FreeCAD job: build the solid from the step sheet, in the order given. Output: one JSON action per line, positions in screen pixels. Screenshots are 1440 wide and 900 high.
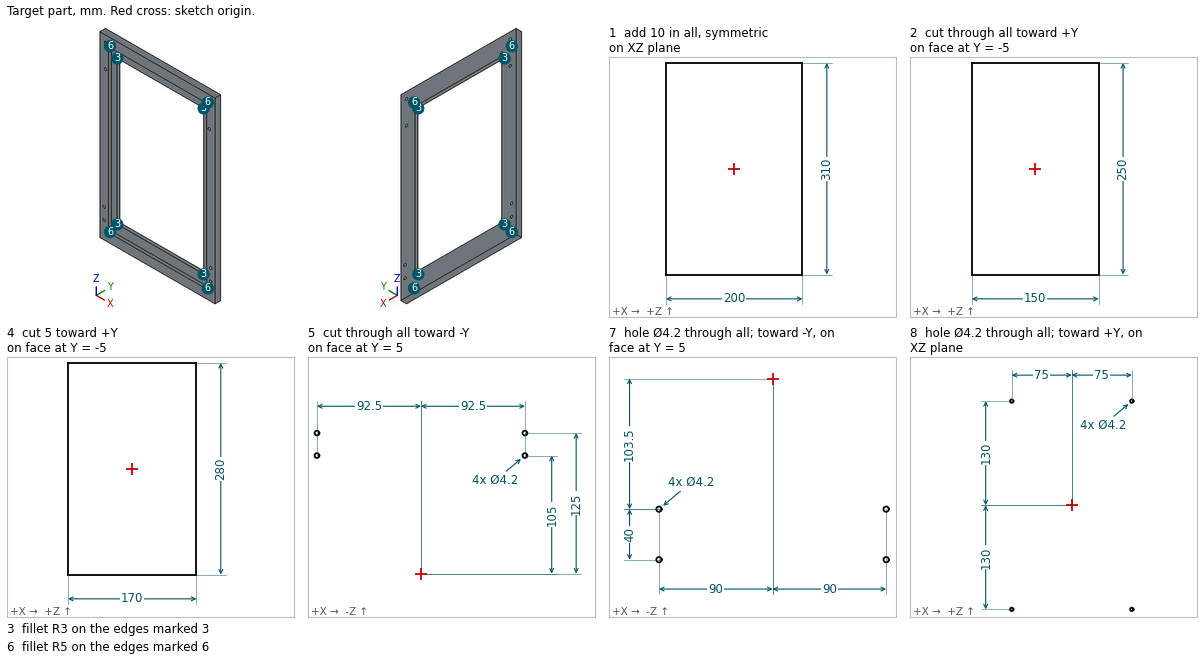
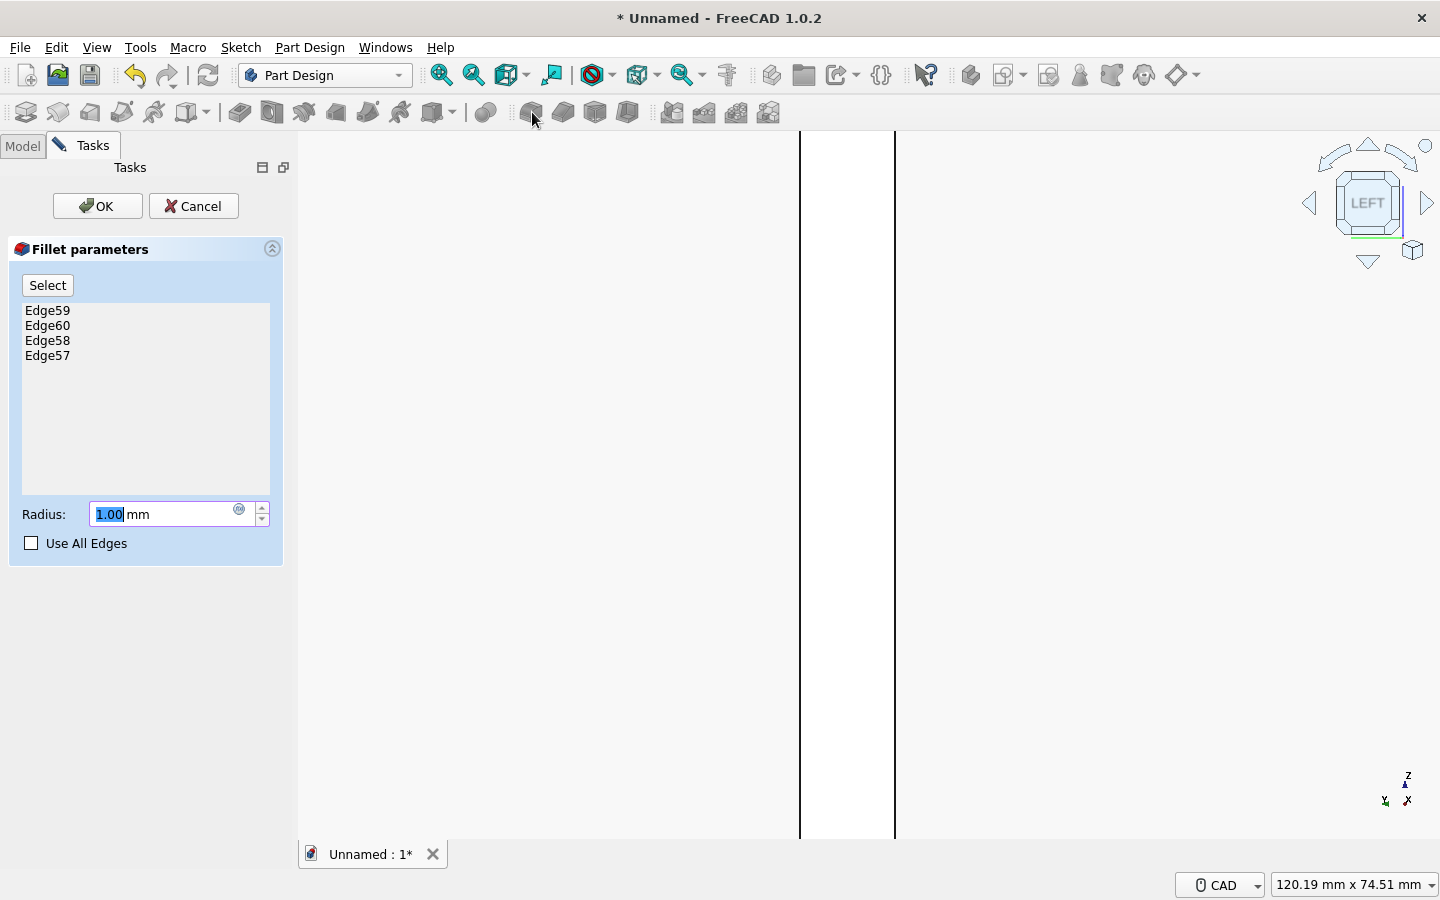
{"action": "type", "text": "5"}
{"action": "key", "text": "Tab"}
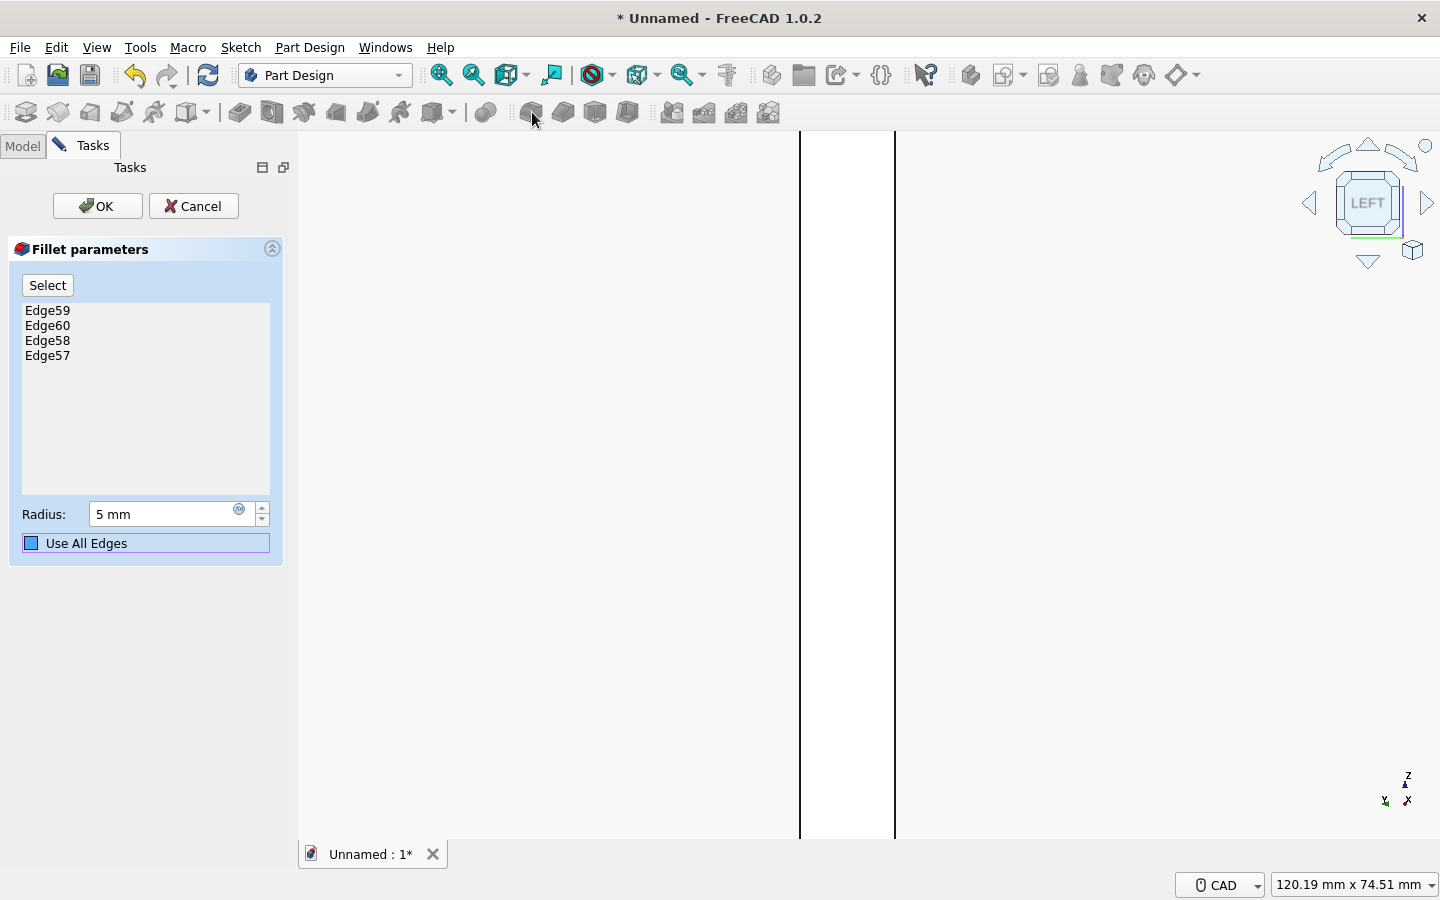
{"action": "left_click", "coordinate": [98, 206]}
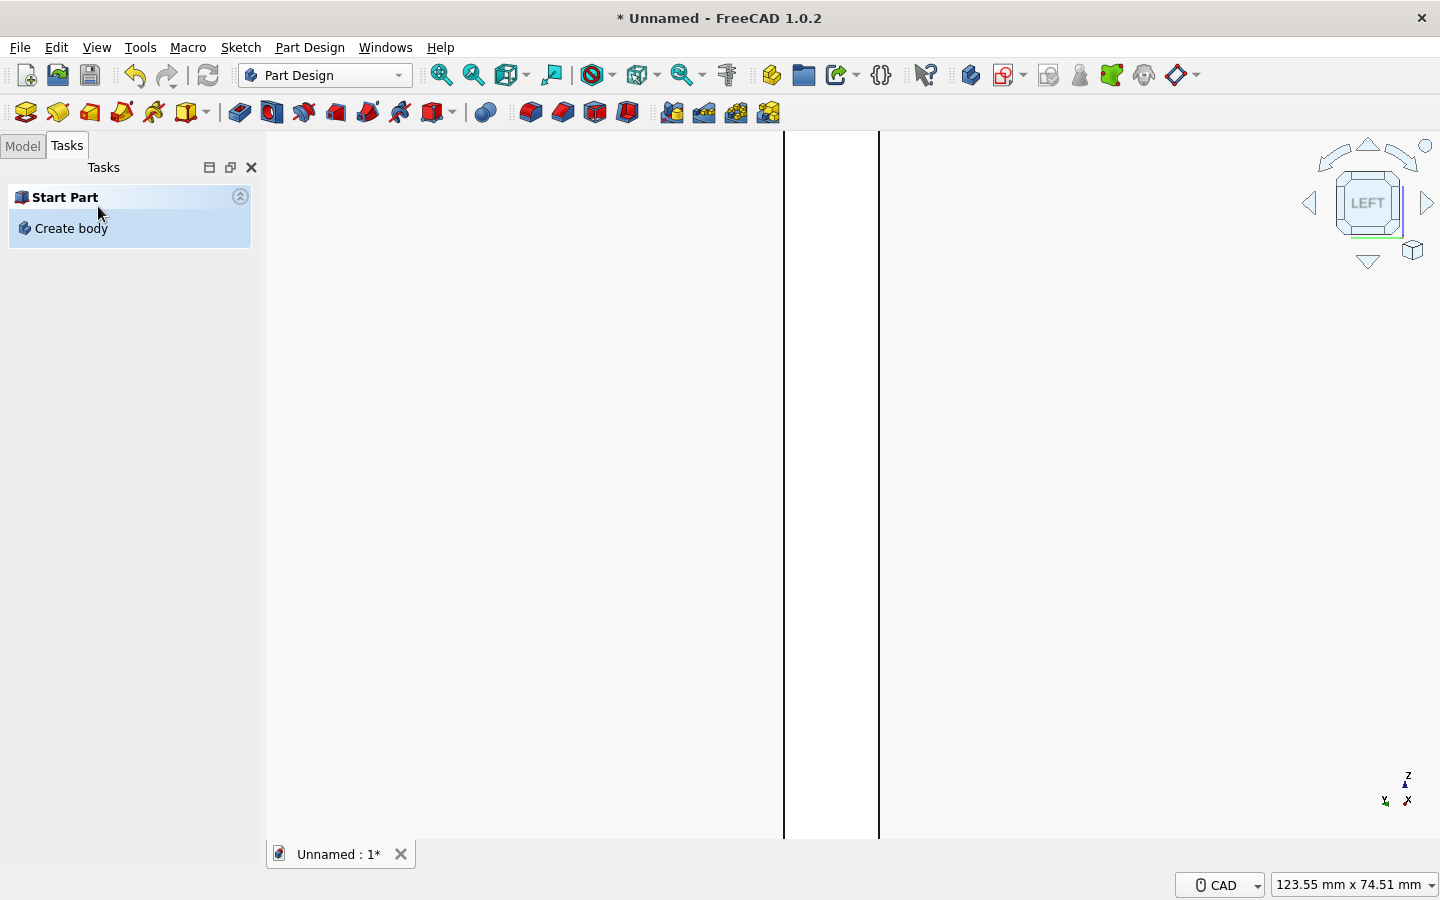
{"action": "key", "text": "v f"}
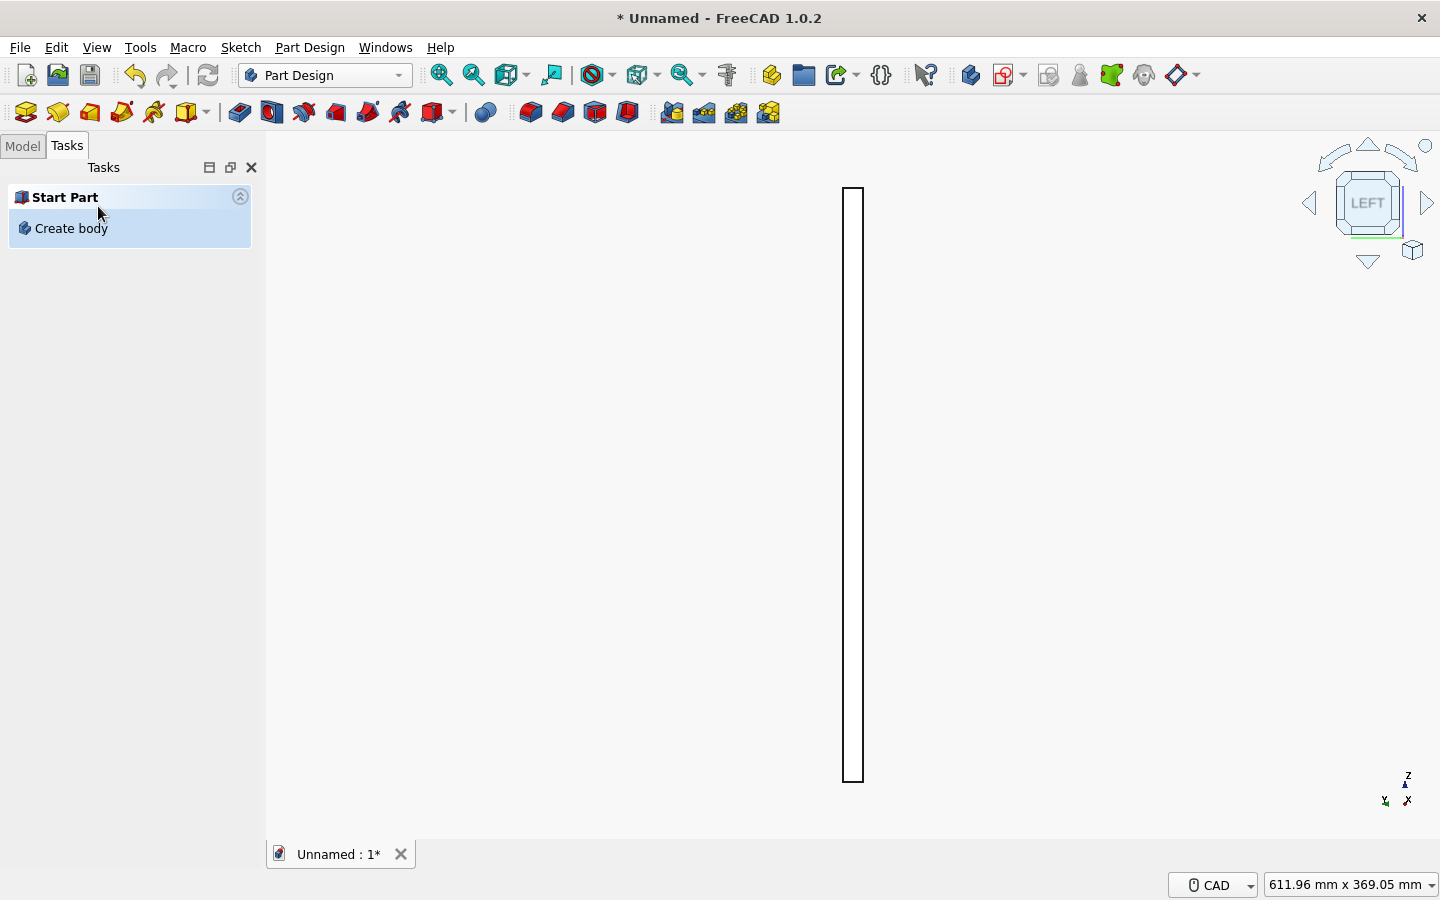
{"action": "key", "text": "4"}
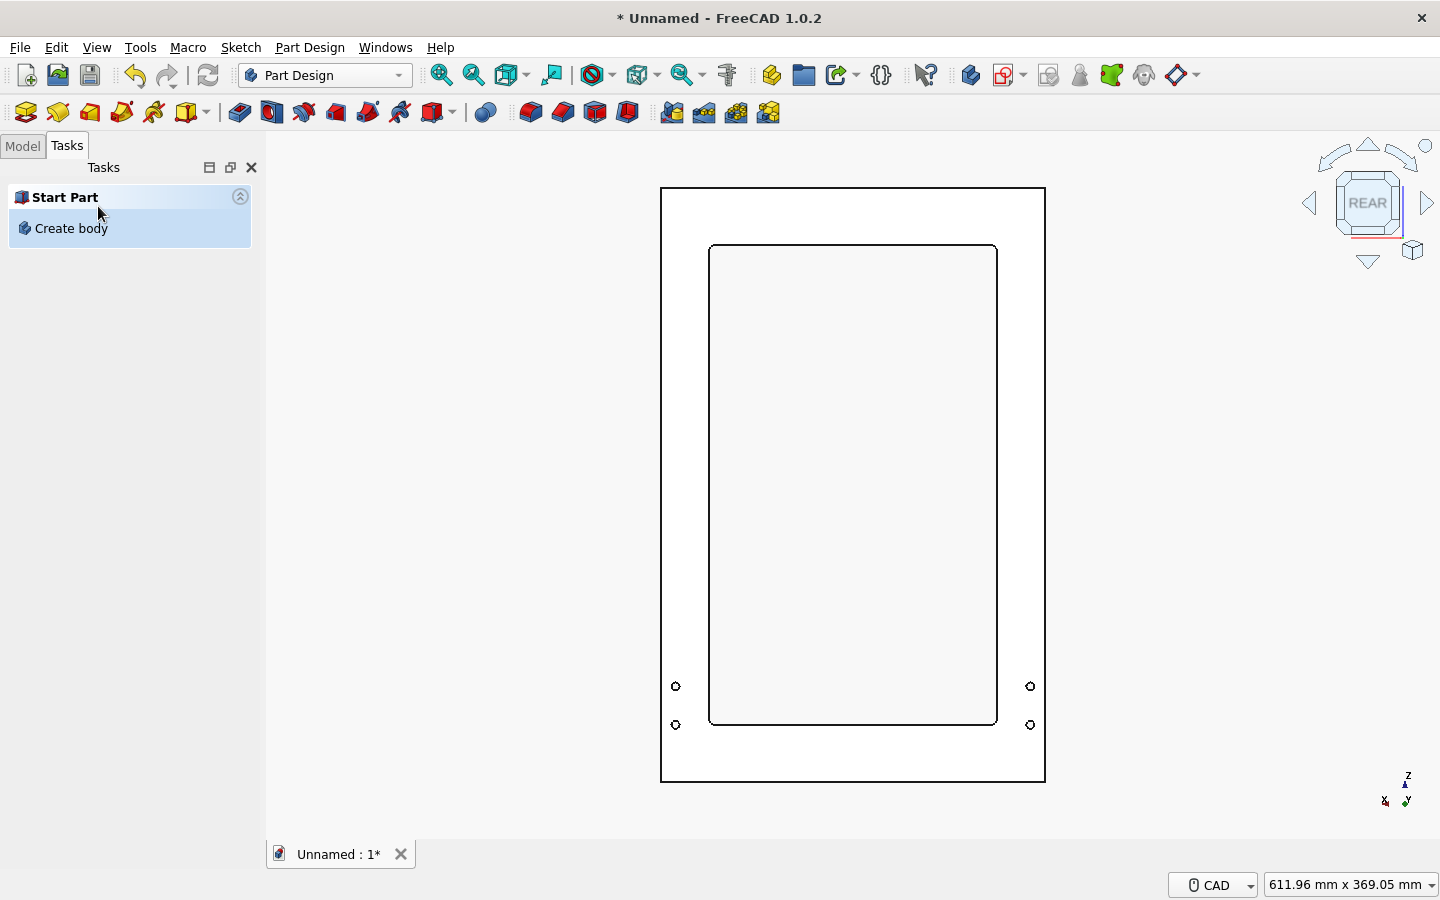
{"action": "left_click", "coordinate": [1017, 229]}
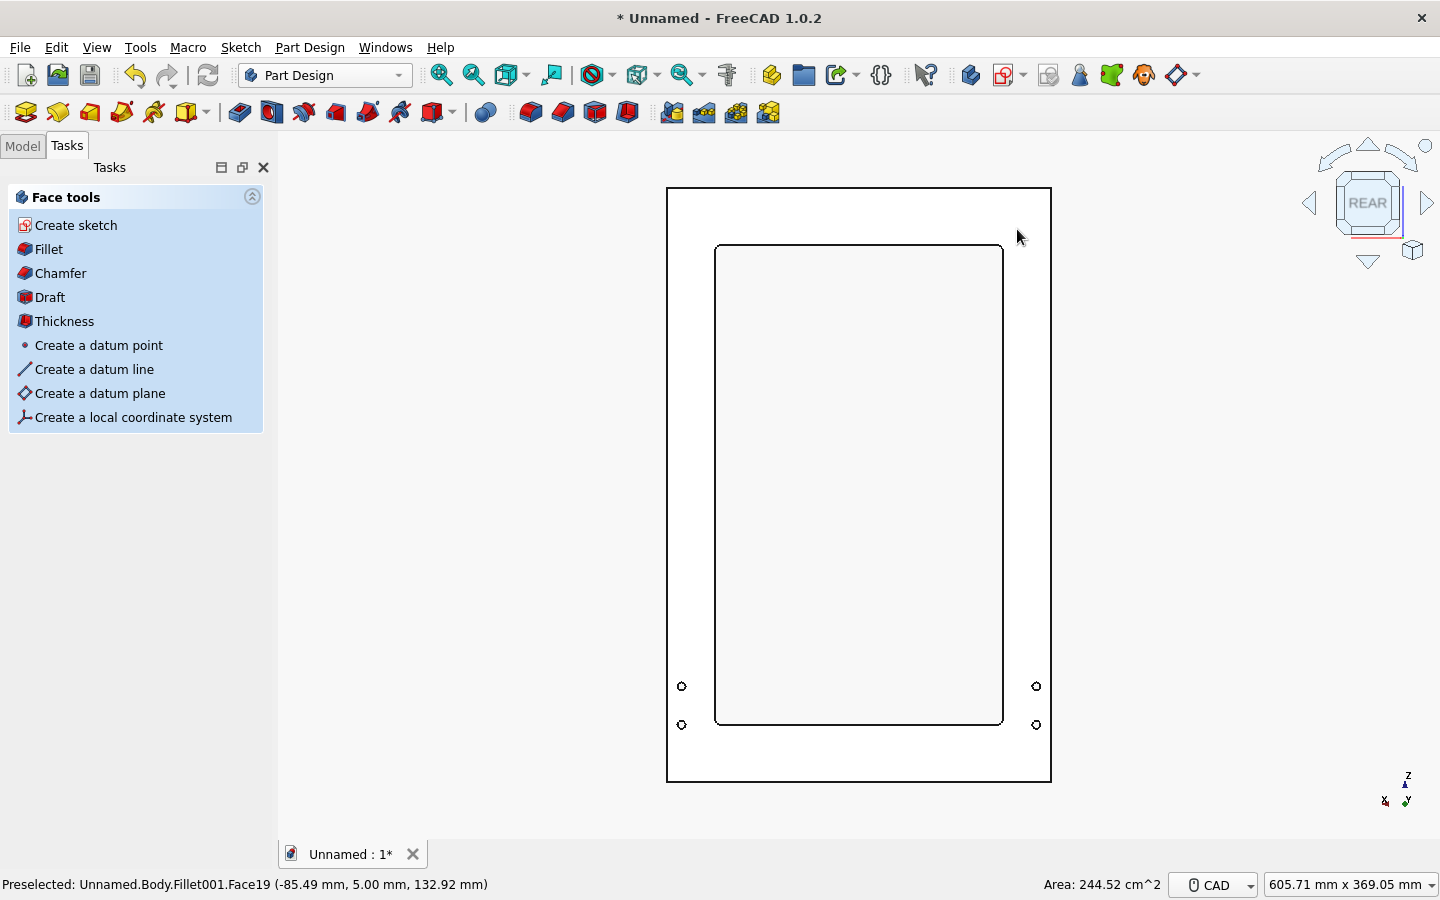
{"action": "left_click", "coordinate": [1004, 76]}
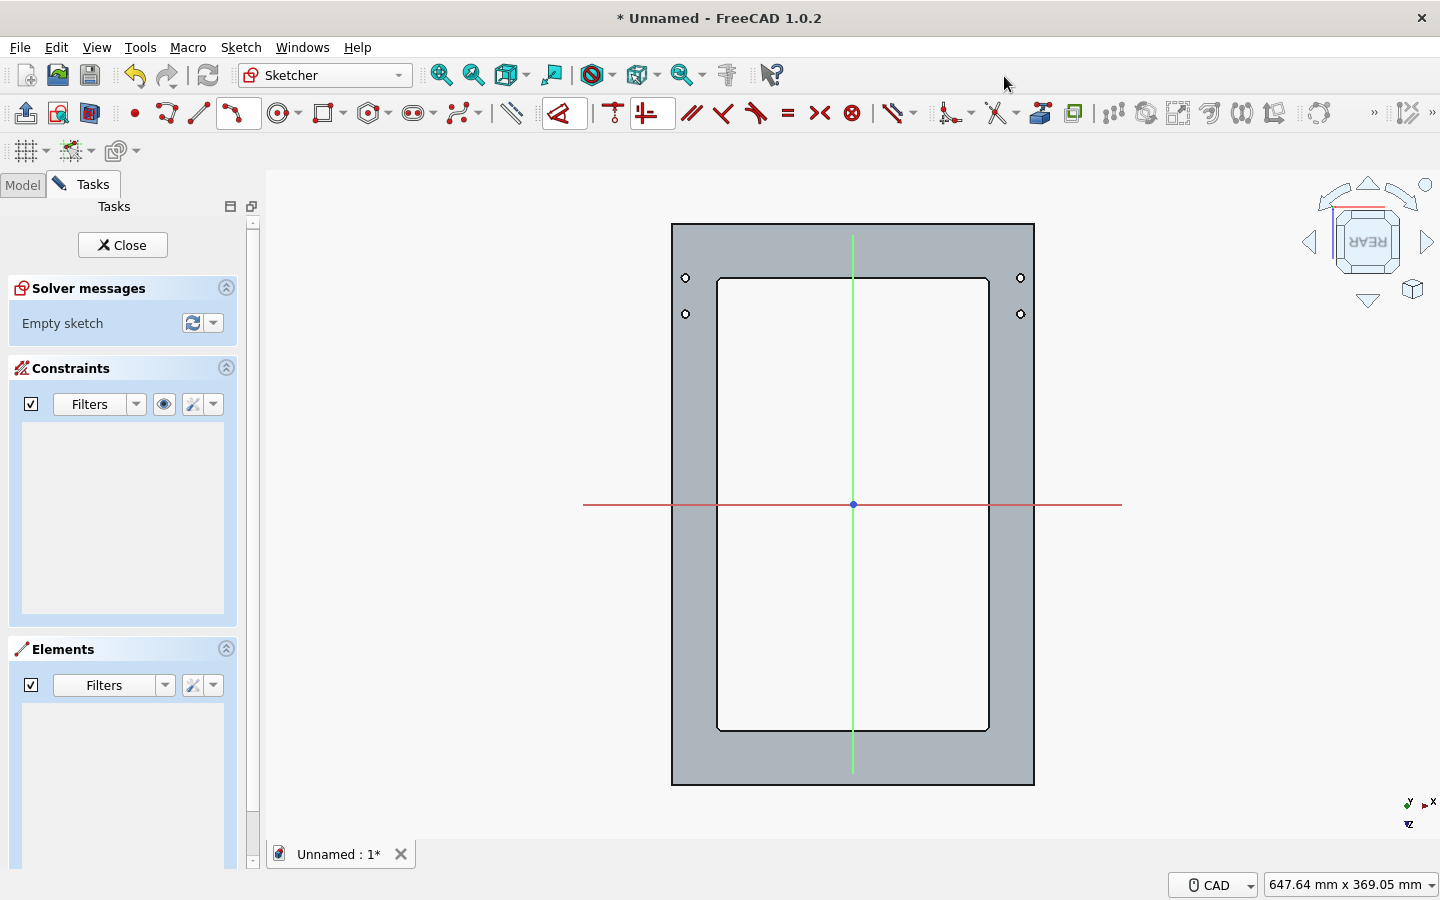
{"action": "scroll", "coordinate": [992, 811], "scroll_direction": "up", "scroll_amount": 2}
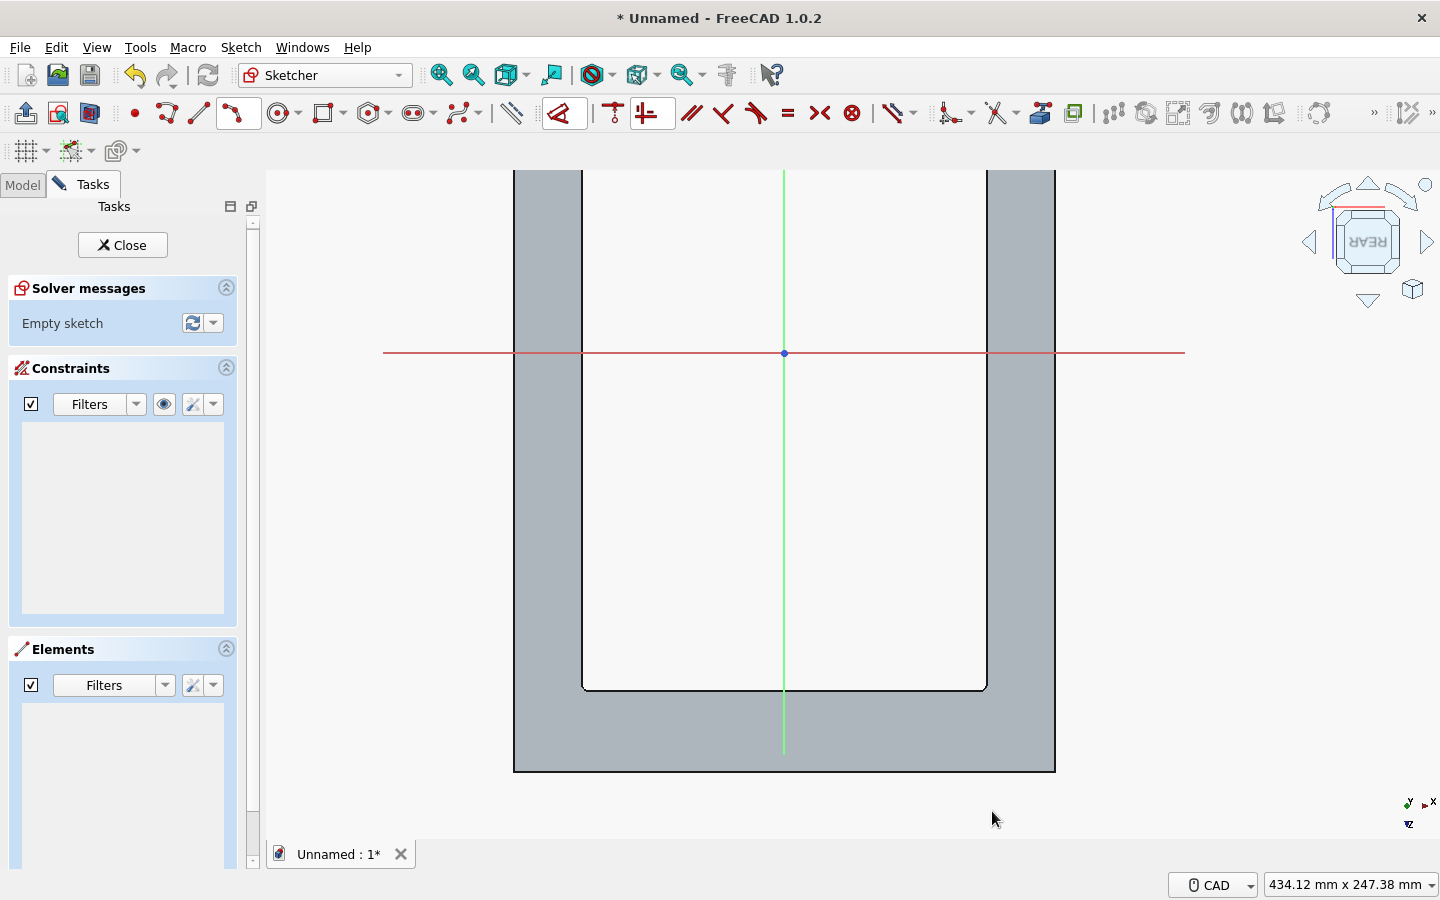
{"action": "key", "text": "g c"}